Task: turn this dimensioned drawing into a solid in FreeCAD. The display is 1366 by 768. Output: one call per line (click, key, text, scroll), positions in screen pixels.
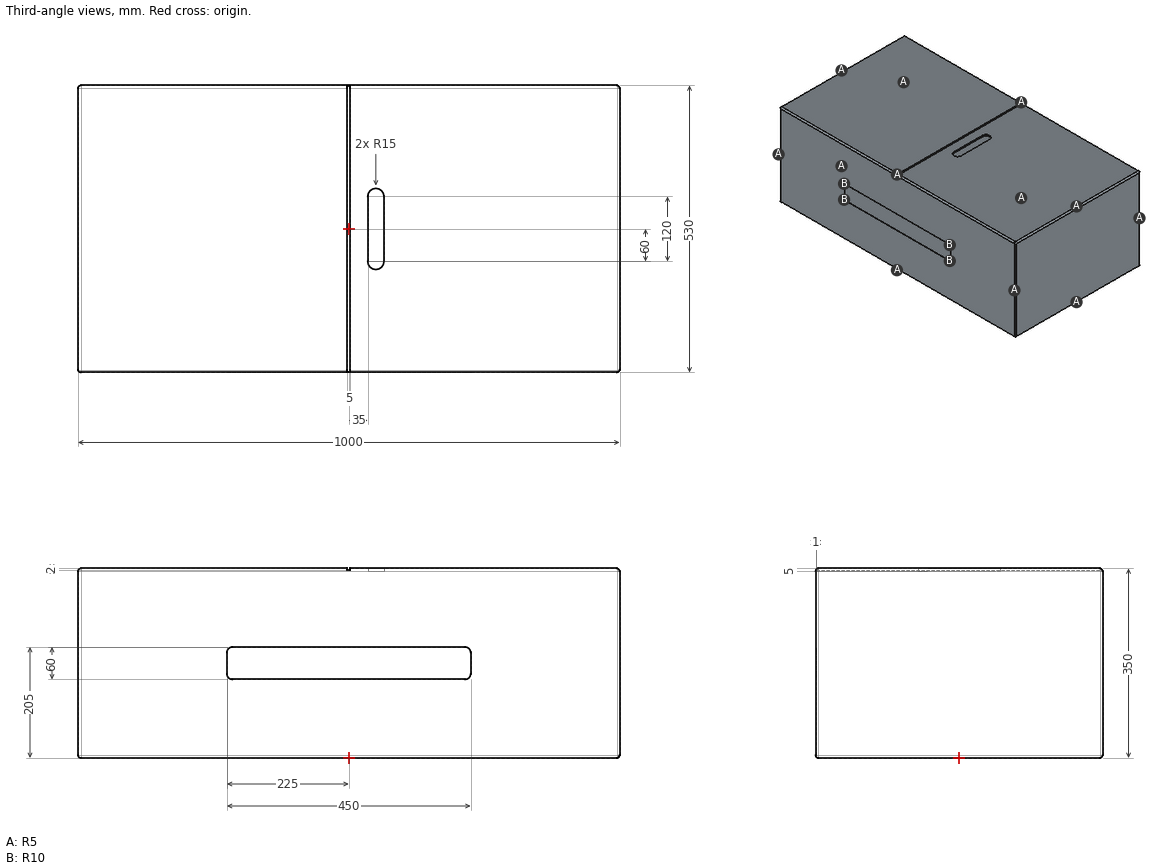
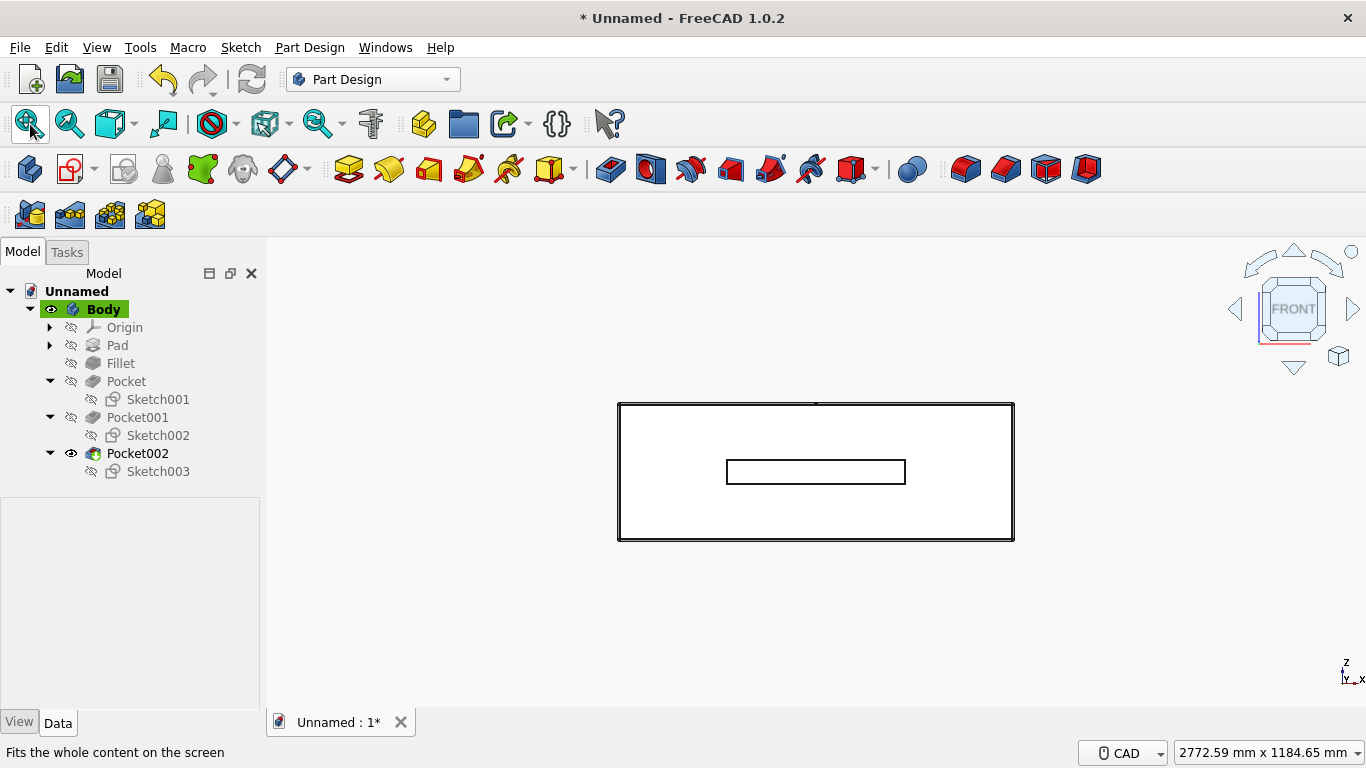
click(30, 124)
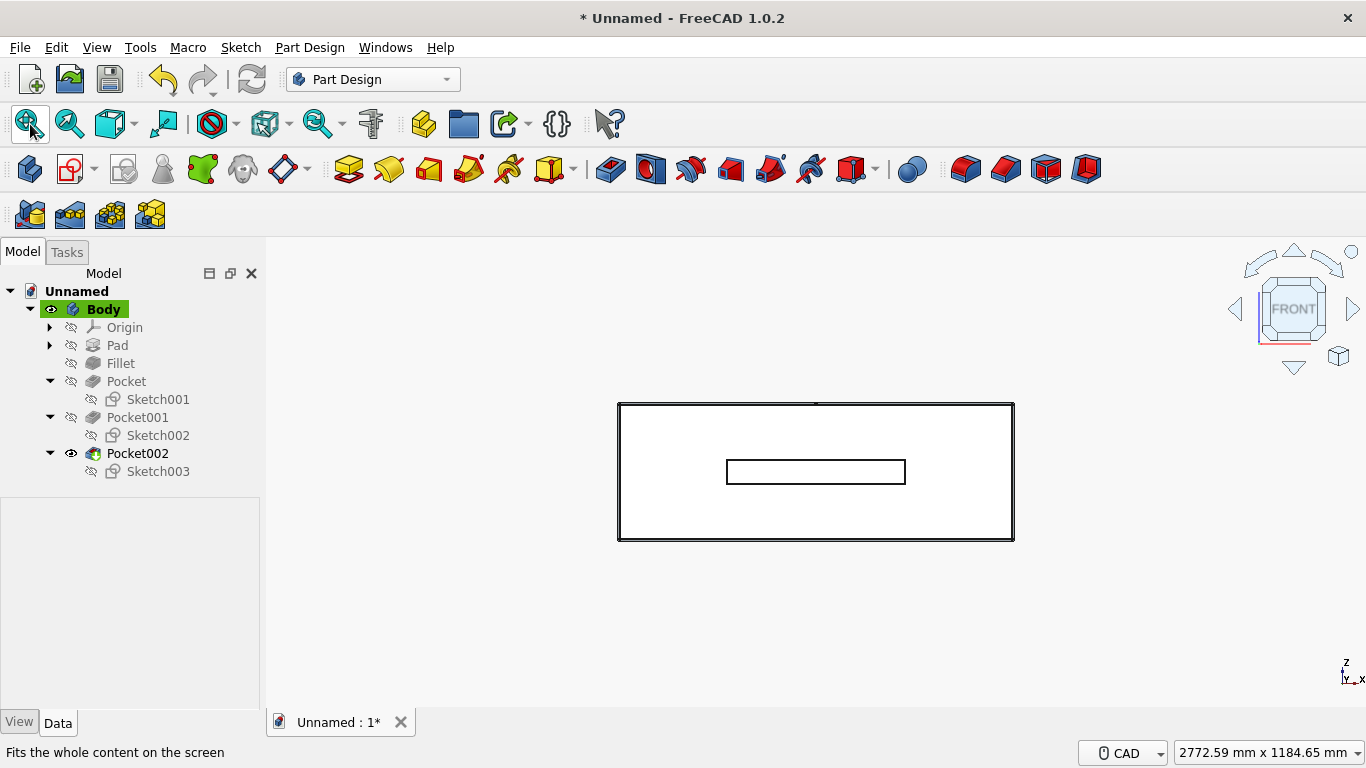
scroll(905, 459, up, 15)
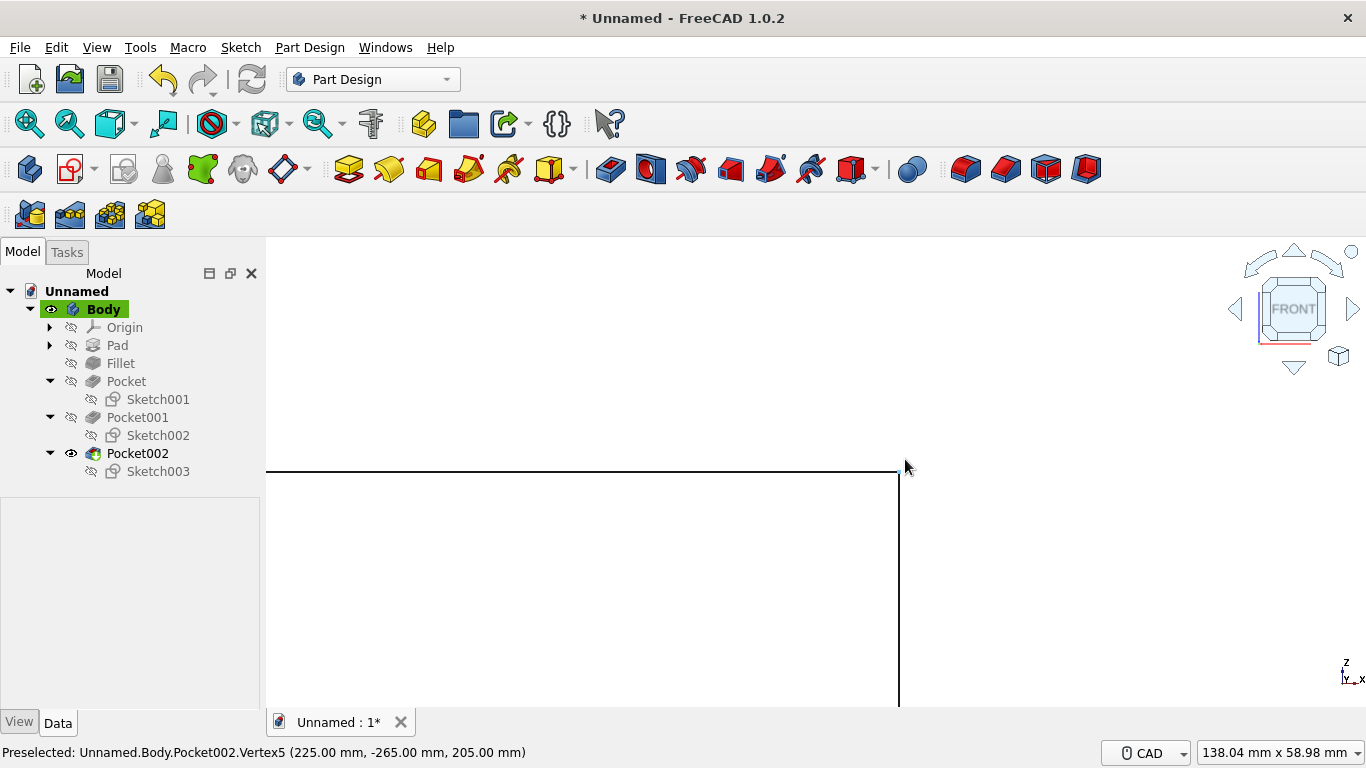
scroll(899, 471, up, 9)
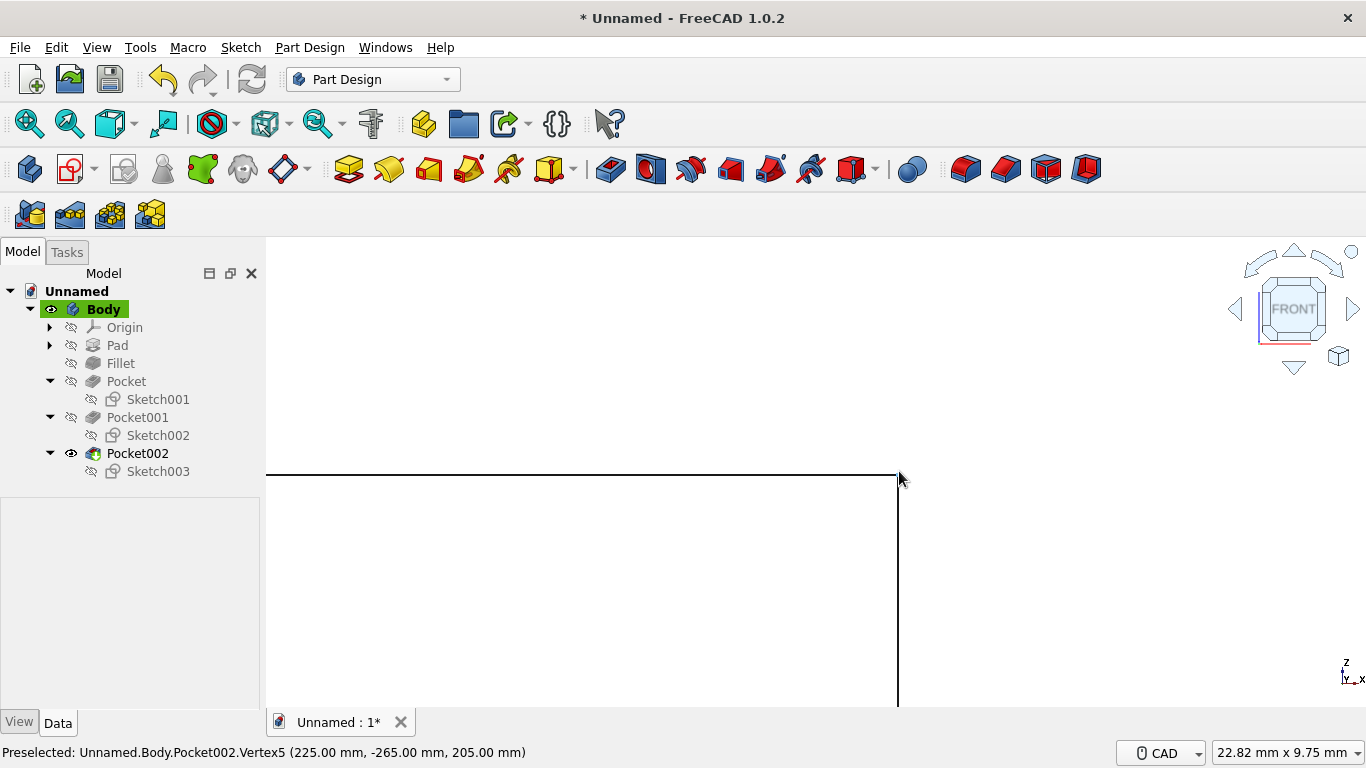
click(30, 124)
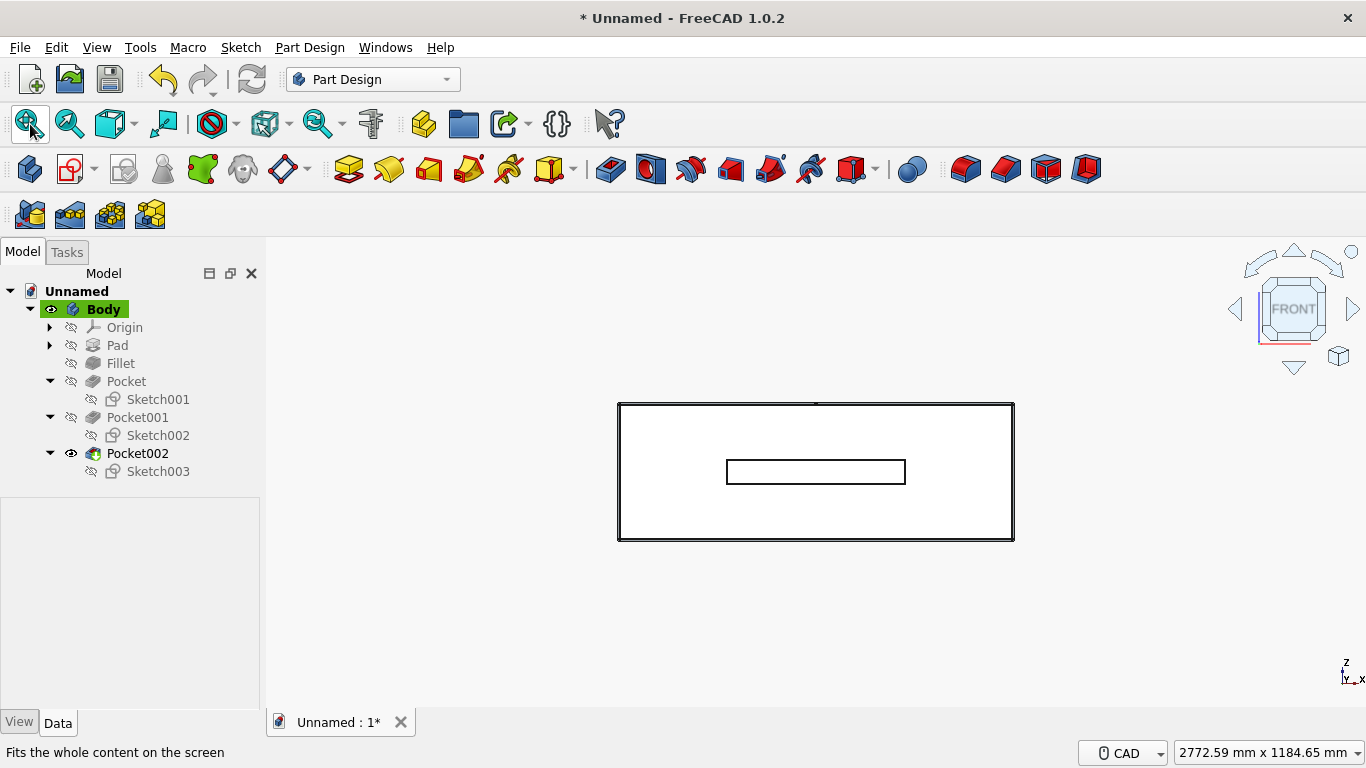
key(3)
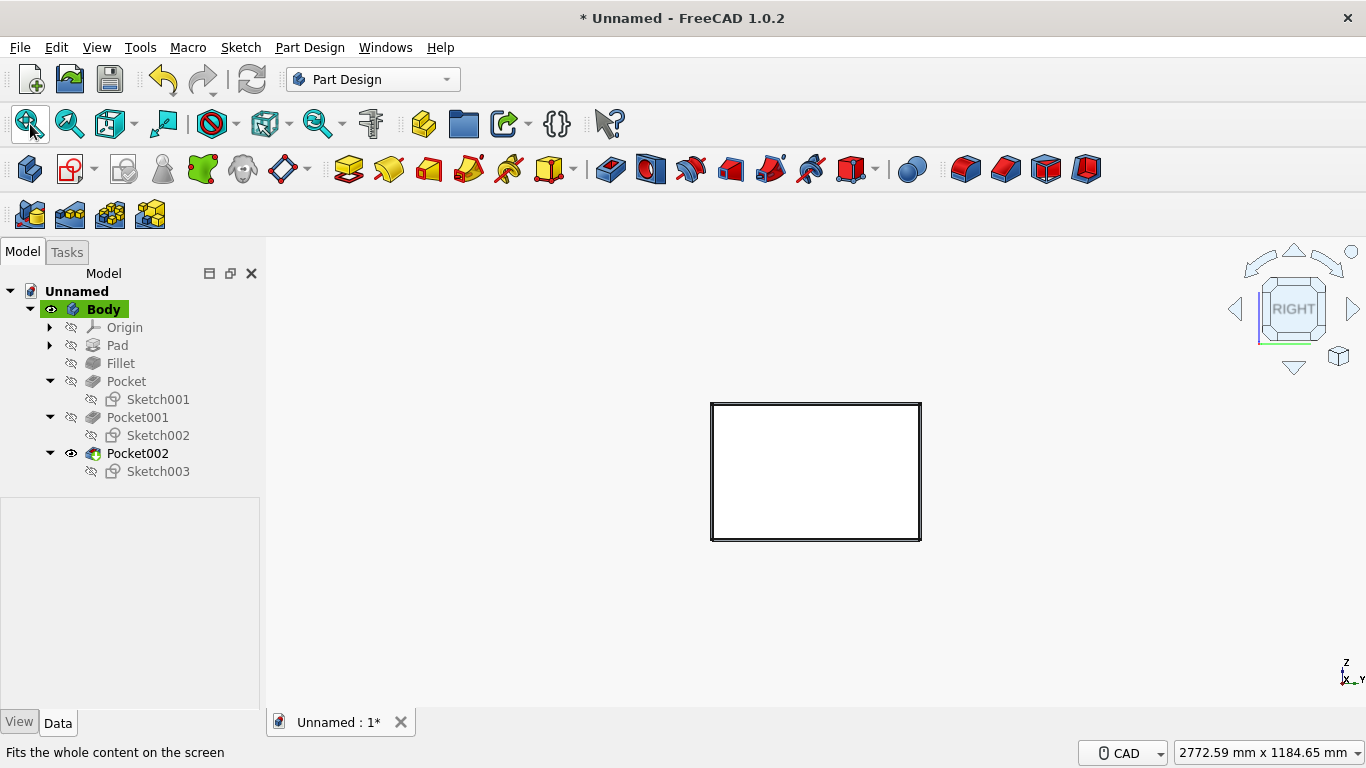
click(30, 124)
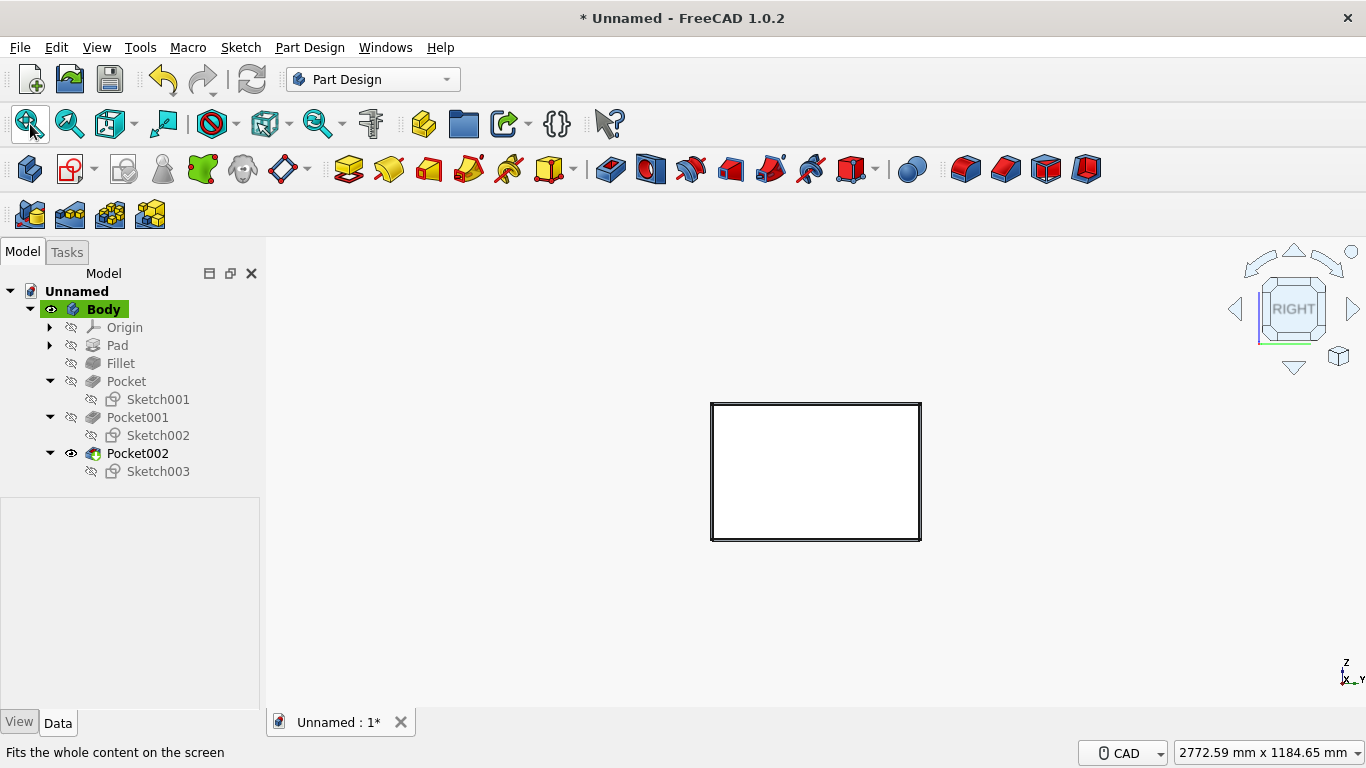
scroll(711, 459, up, 15)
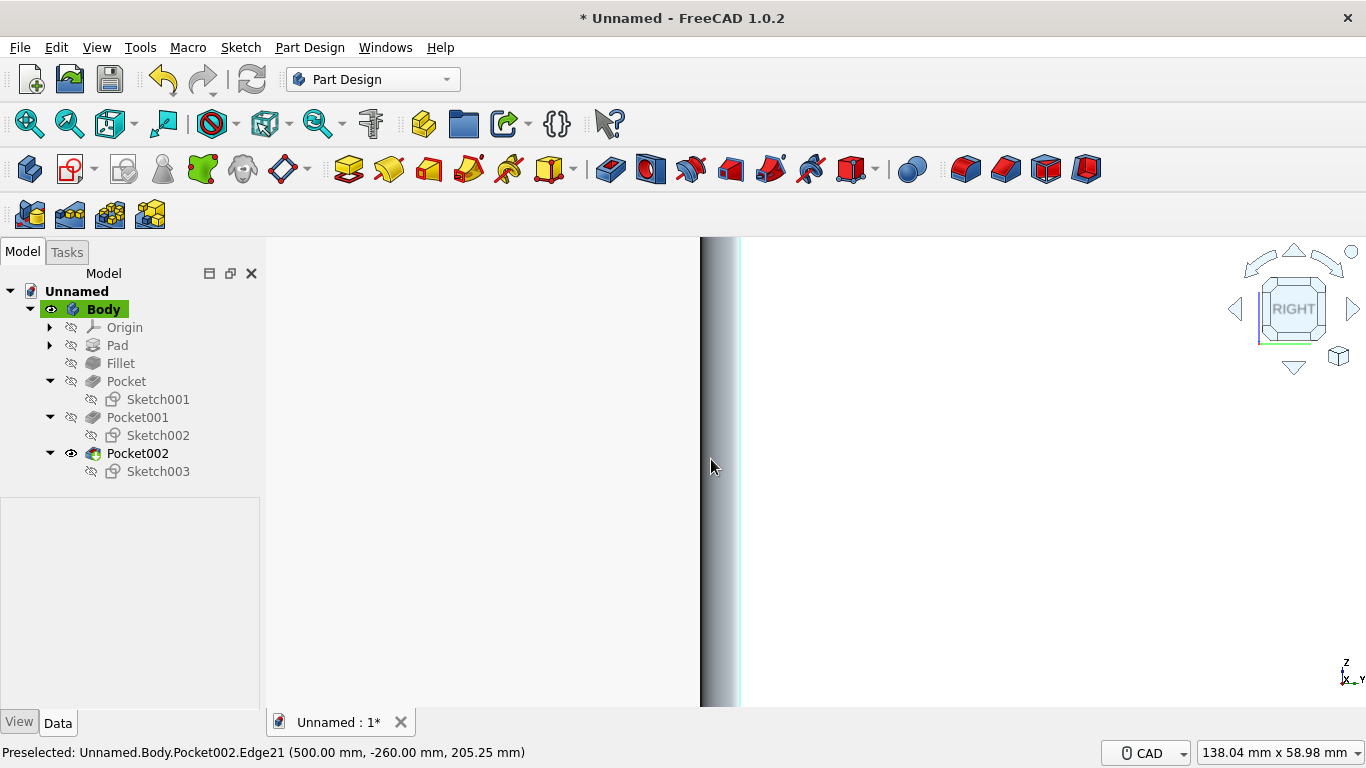
scroll(705, 471, up, 9)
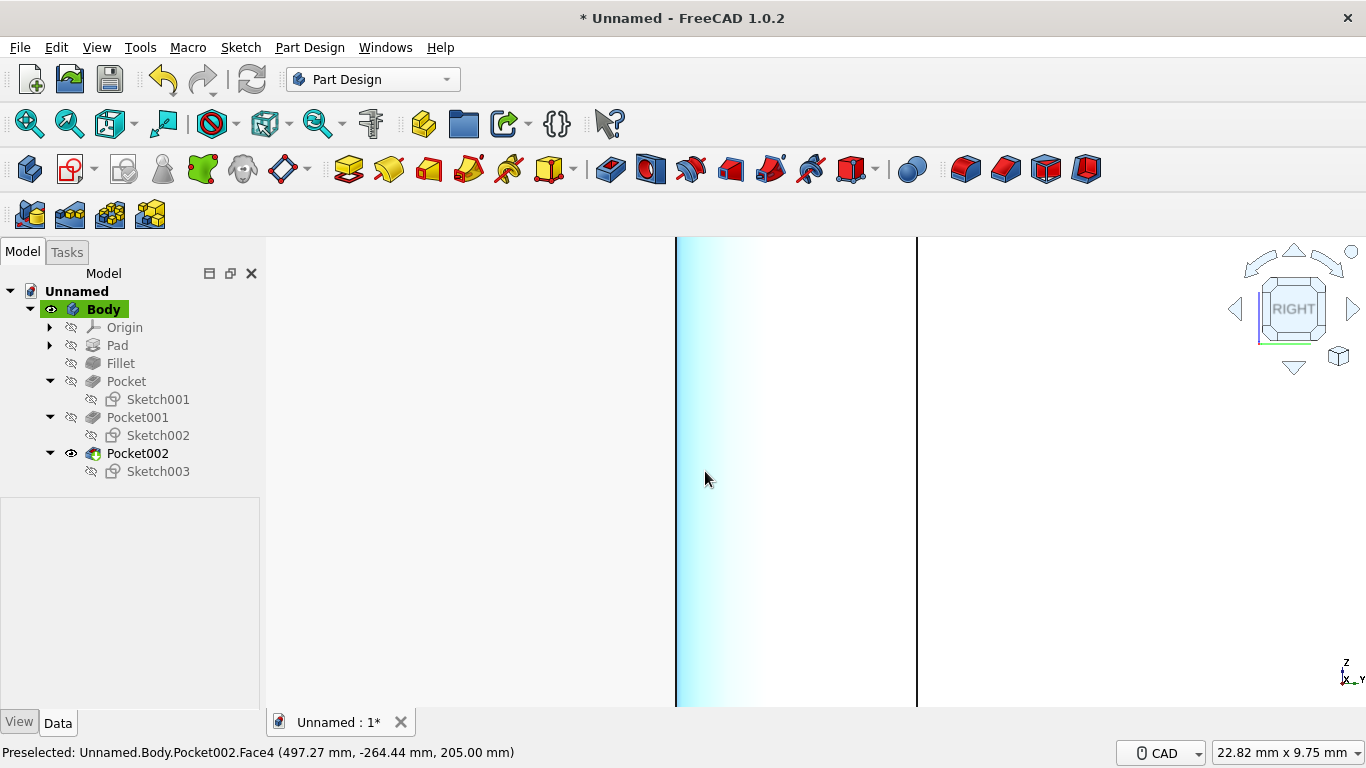
click(30, 124)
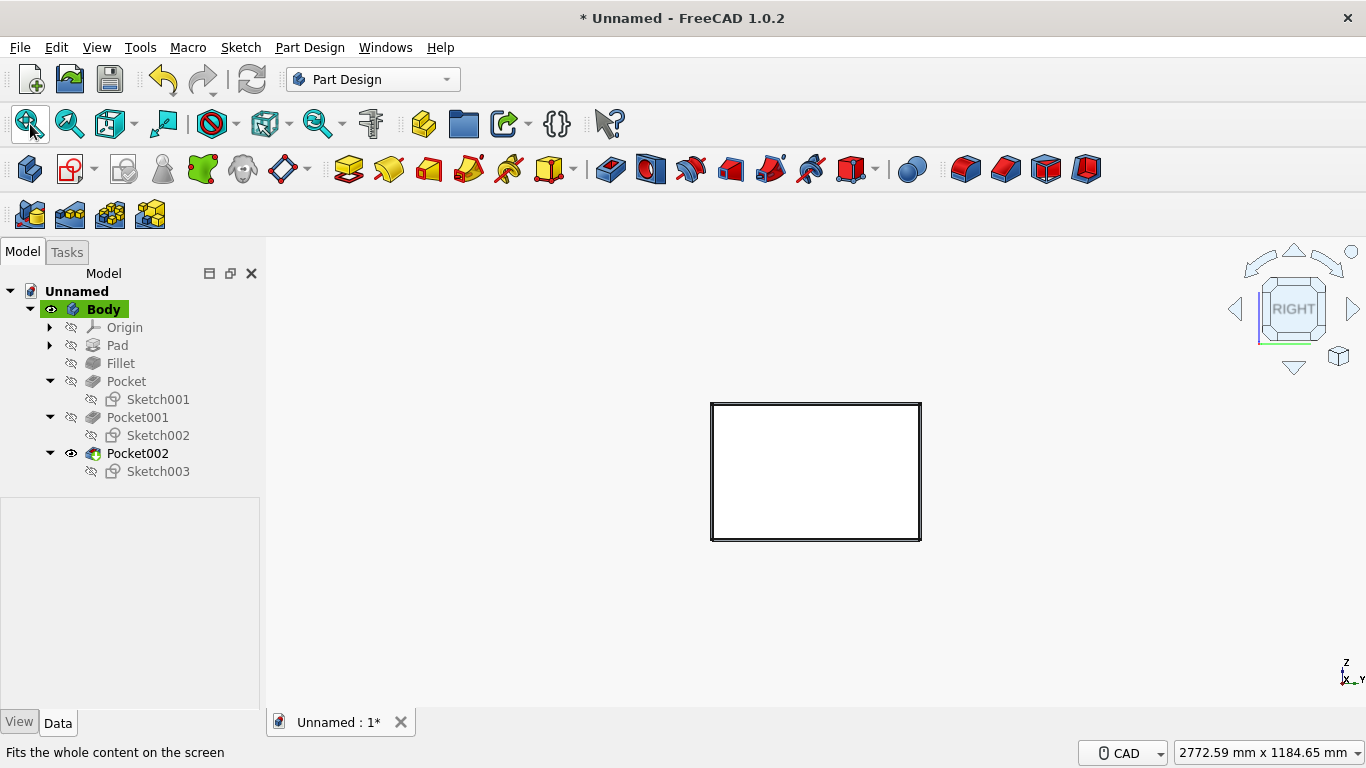
key(5)